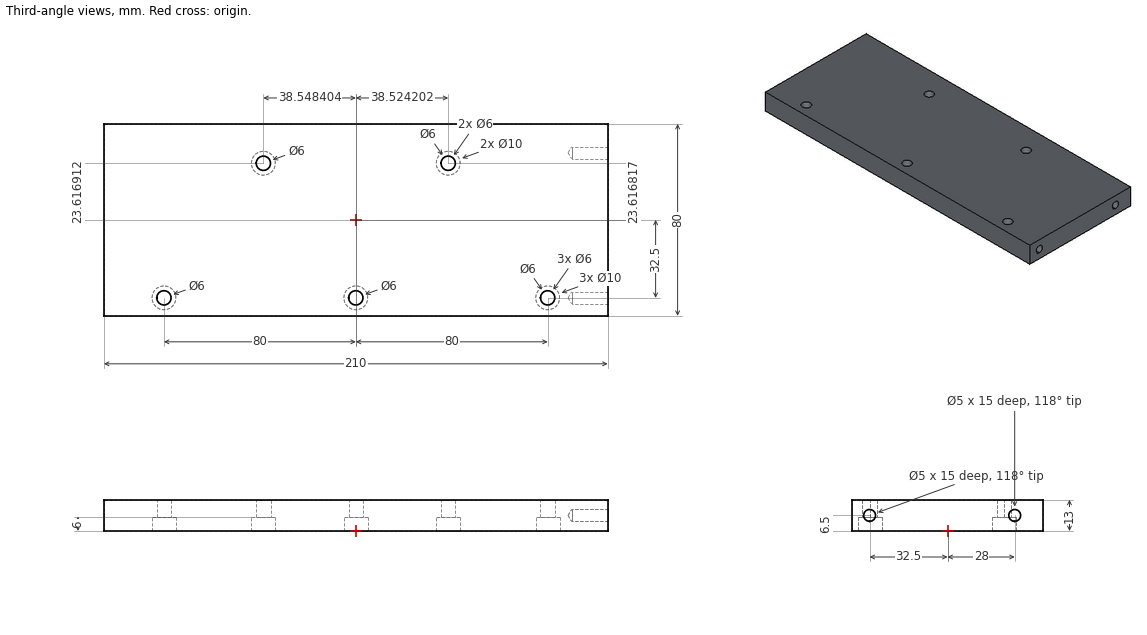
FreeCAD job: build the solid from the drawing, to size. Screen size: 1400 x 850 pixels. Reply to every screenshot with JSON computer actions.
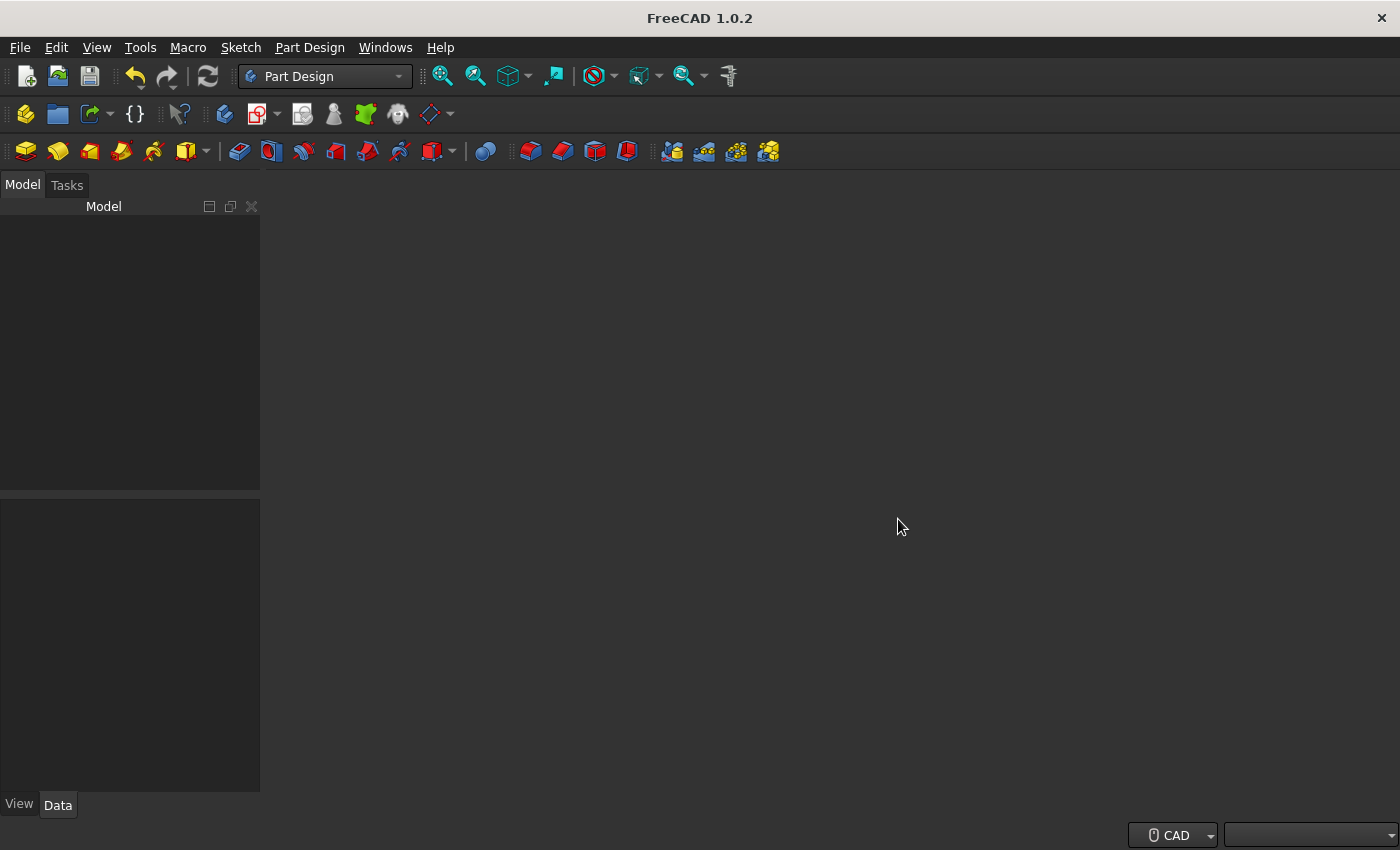
{"action": "left_click", "coordinate": [26, 76]}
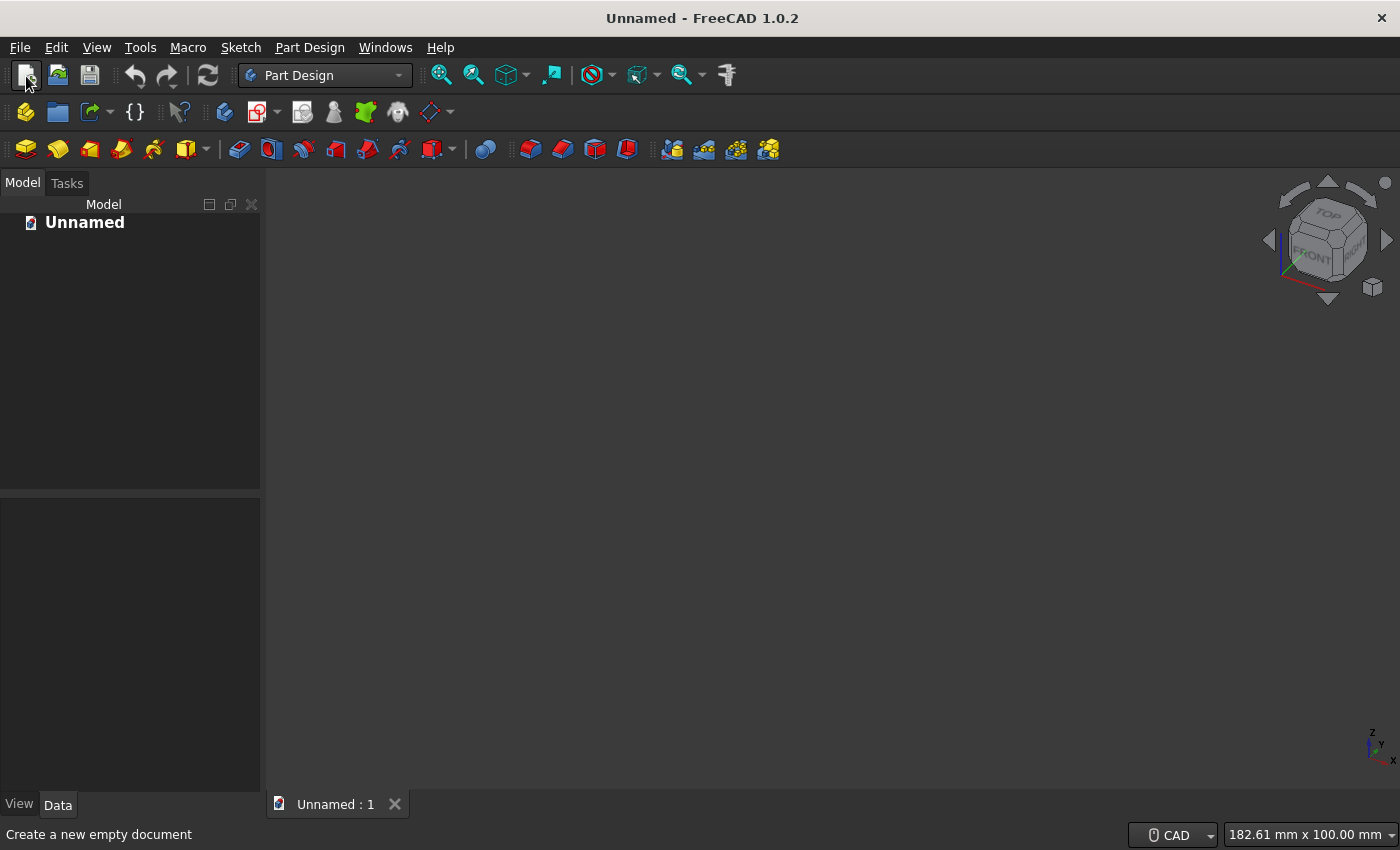
{"action": "left_click", "coordinate": [258, 112]}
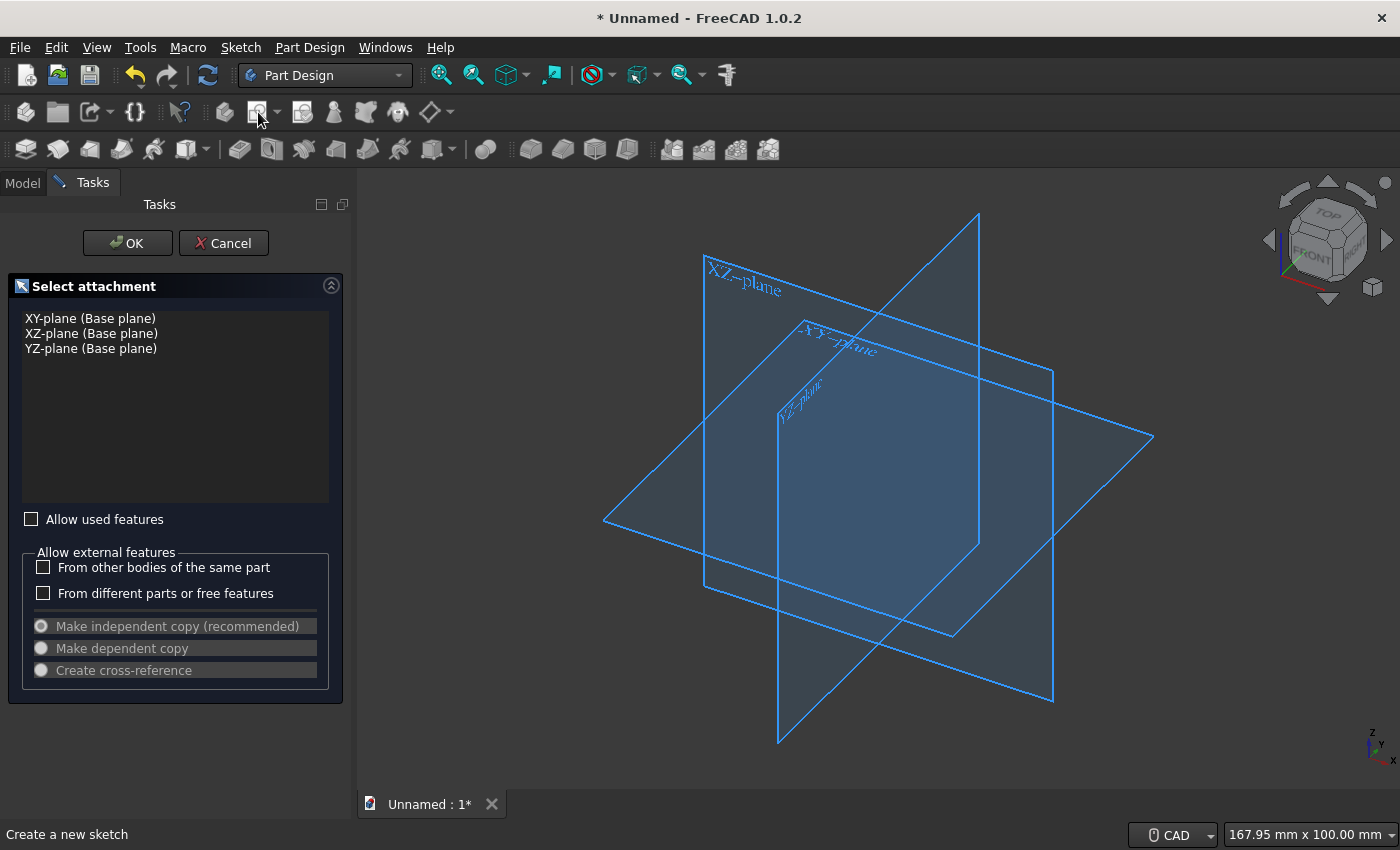
{"action": "left_click", "coordinate": [82, 318]}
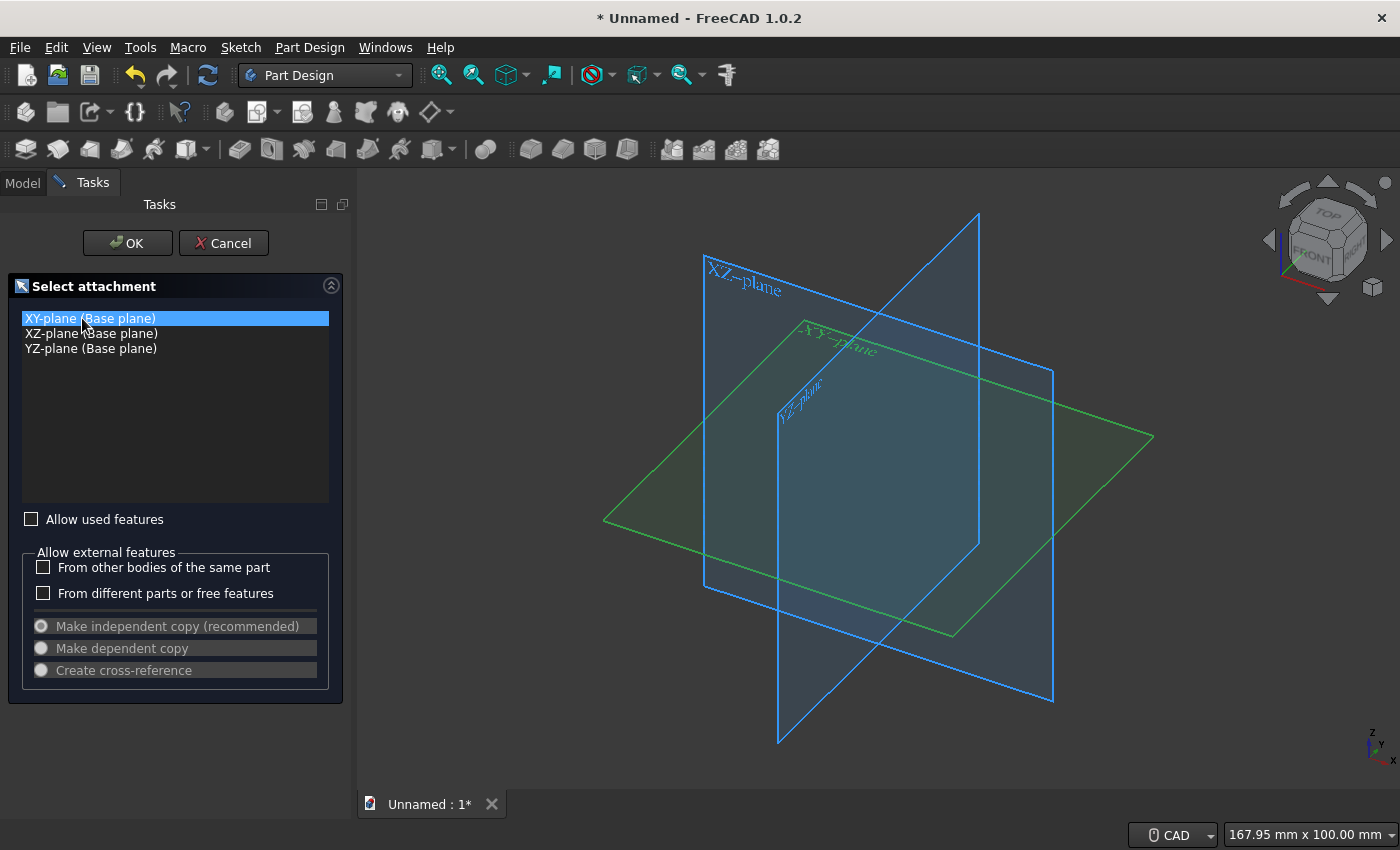
{"action": "left_click", "coordinate": [128, 243]}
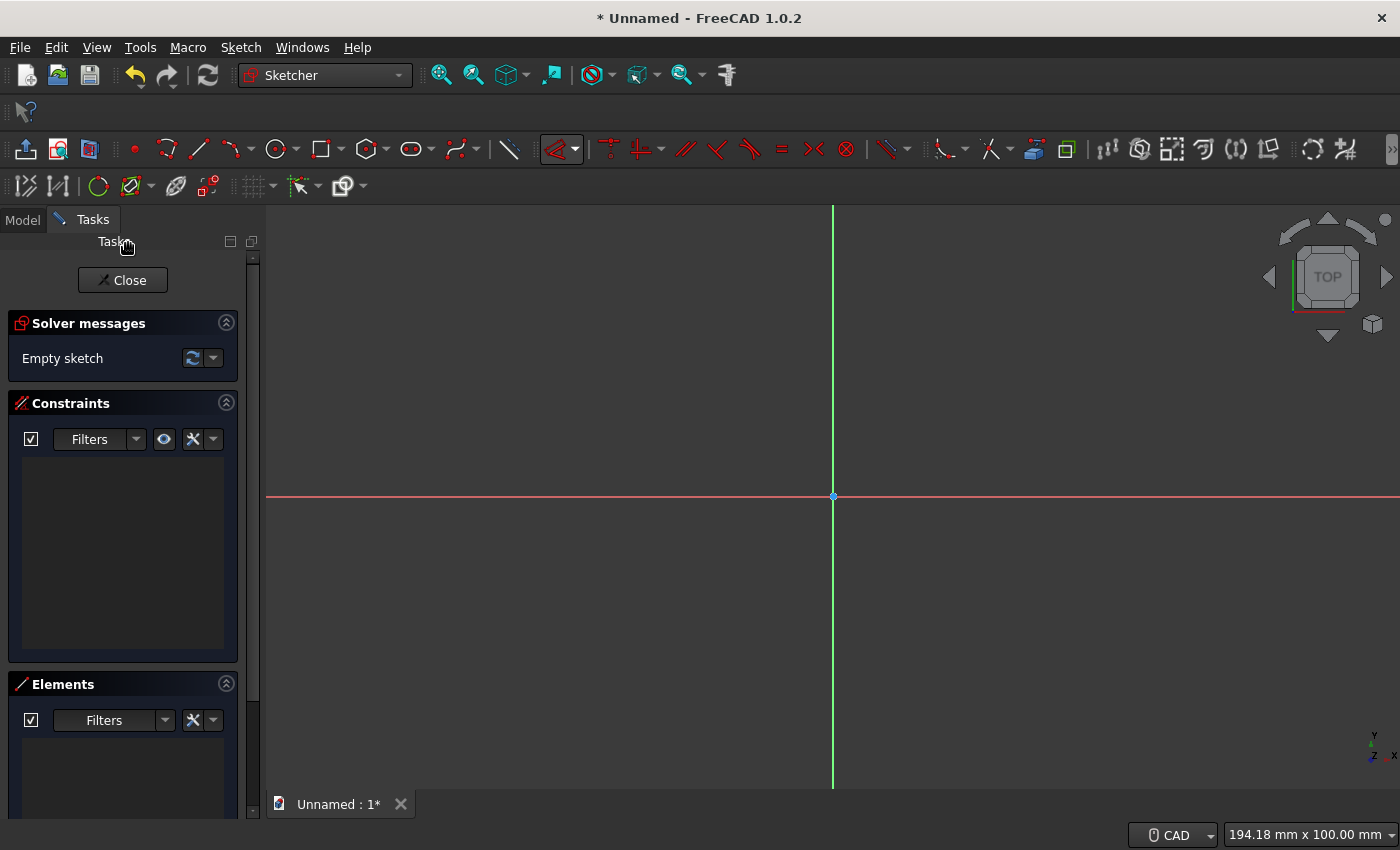
{"action": "scroll", "coordinate": [681, 497], "scroll_direction": "down", "scroll_amount": 3}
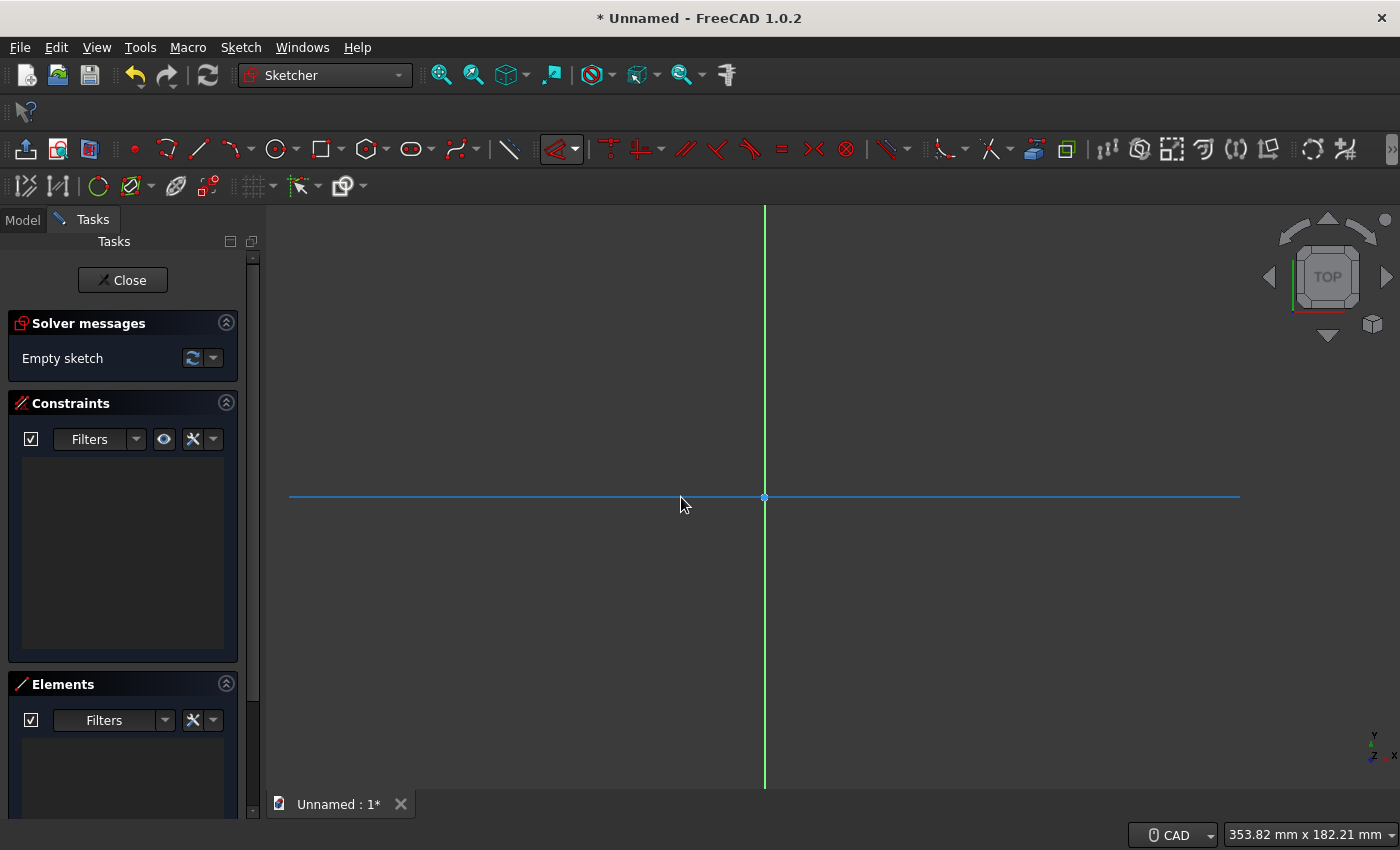
{"action": "key", "text": "g v"}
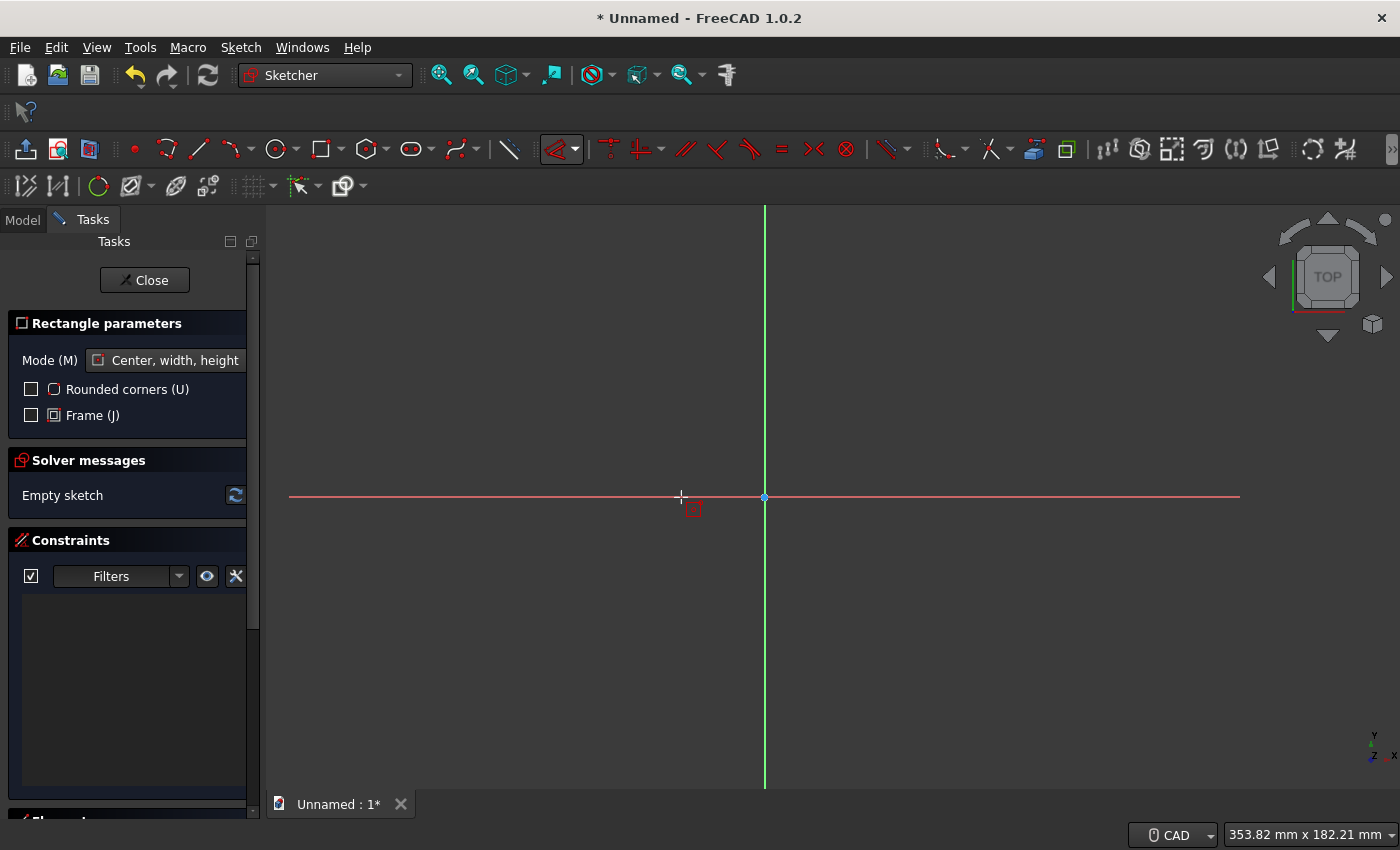
{"action": "left_click", "coordinate": [765, 497]}
{"action": "left_click", "coordinate": [1101, 369]}
{"action": "key", "text": "Escape"}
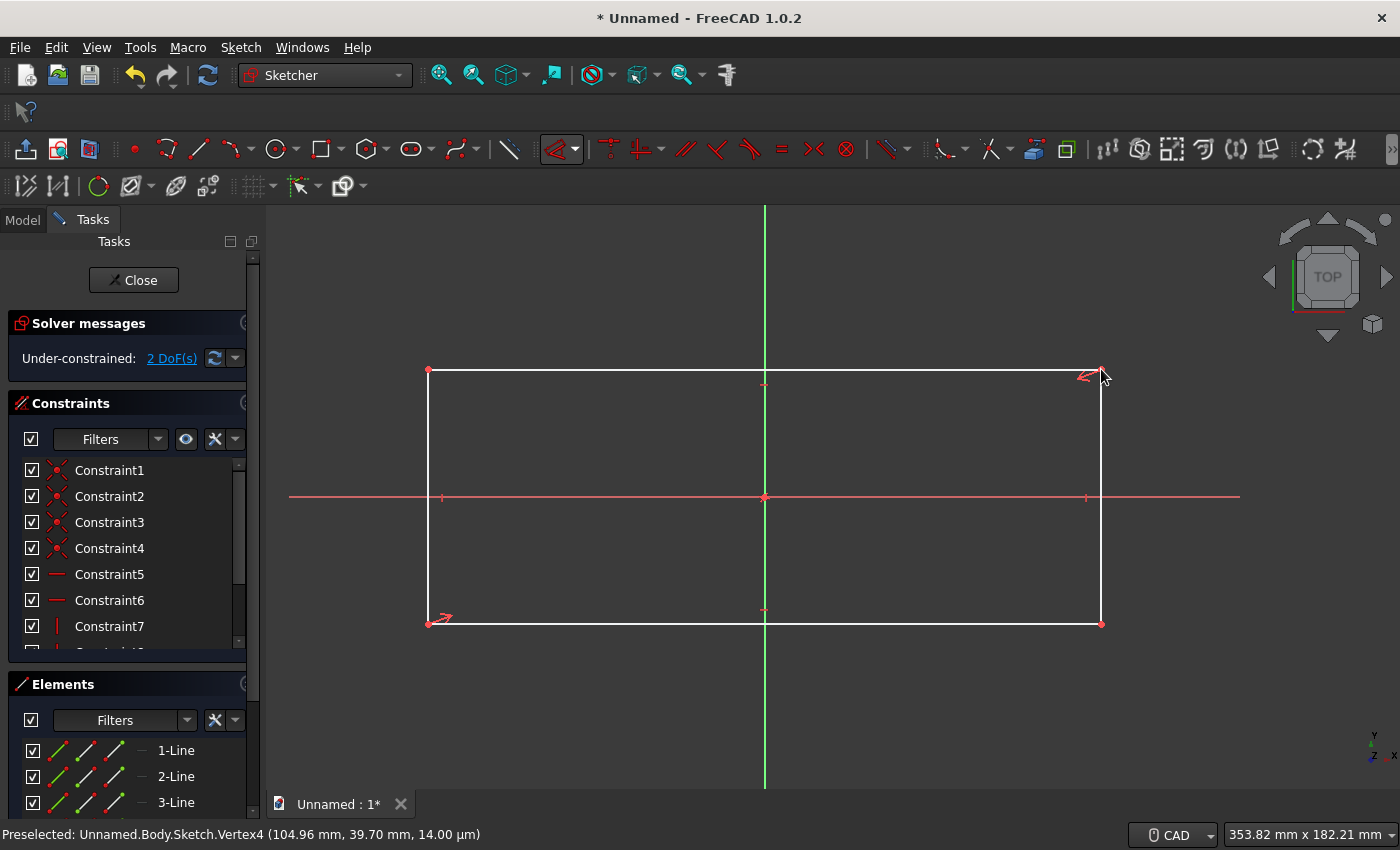
{"action": "key", "text": "d"}